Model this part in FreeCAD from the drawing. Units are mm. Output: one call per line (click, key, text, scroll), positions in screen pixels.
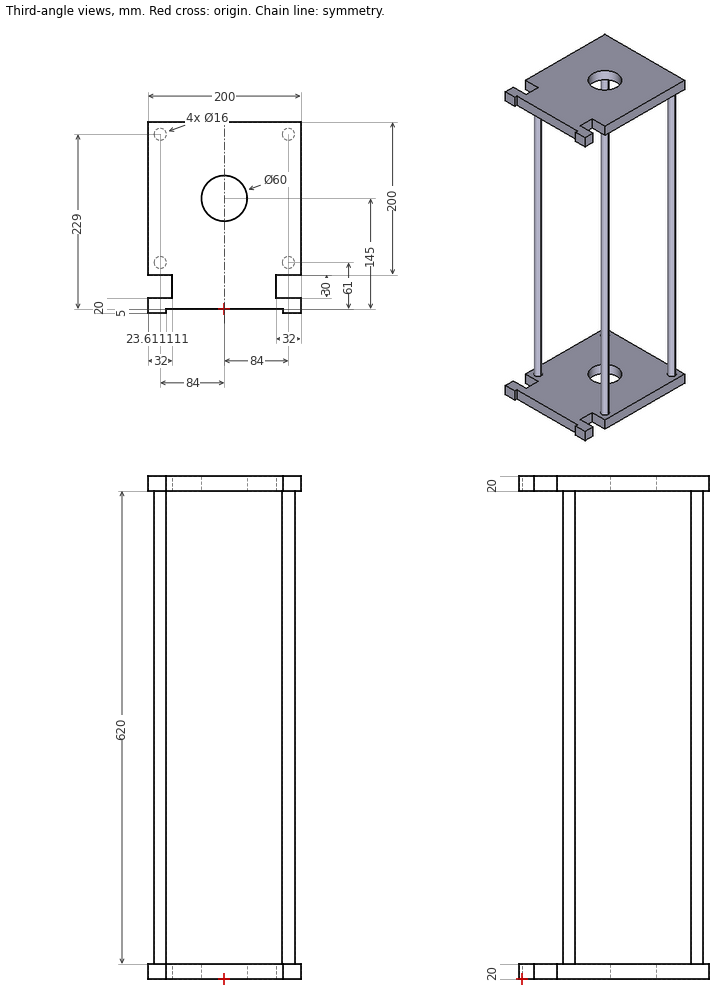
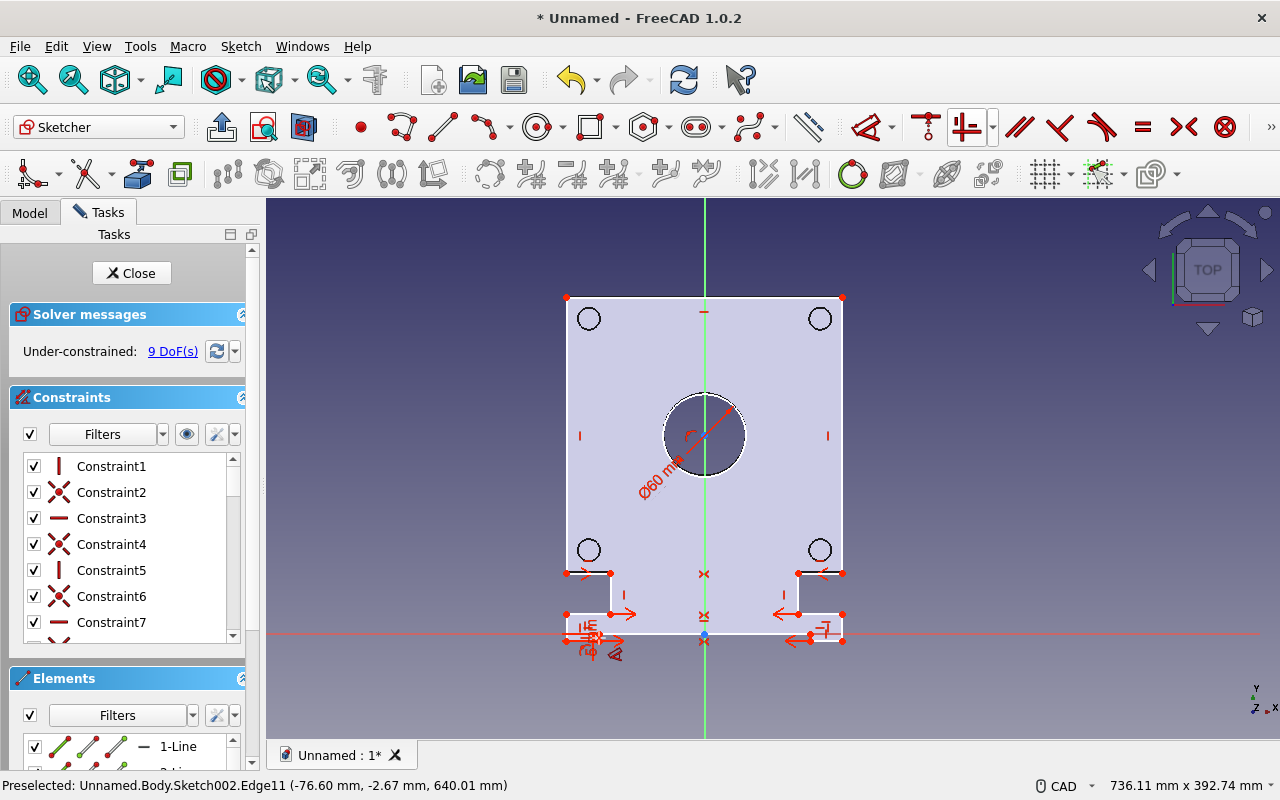
click(798, 602)
click(832, 594)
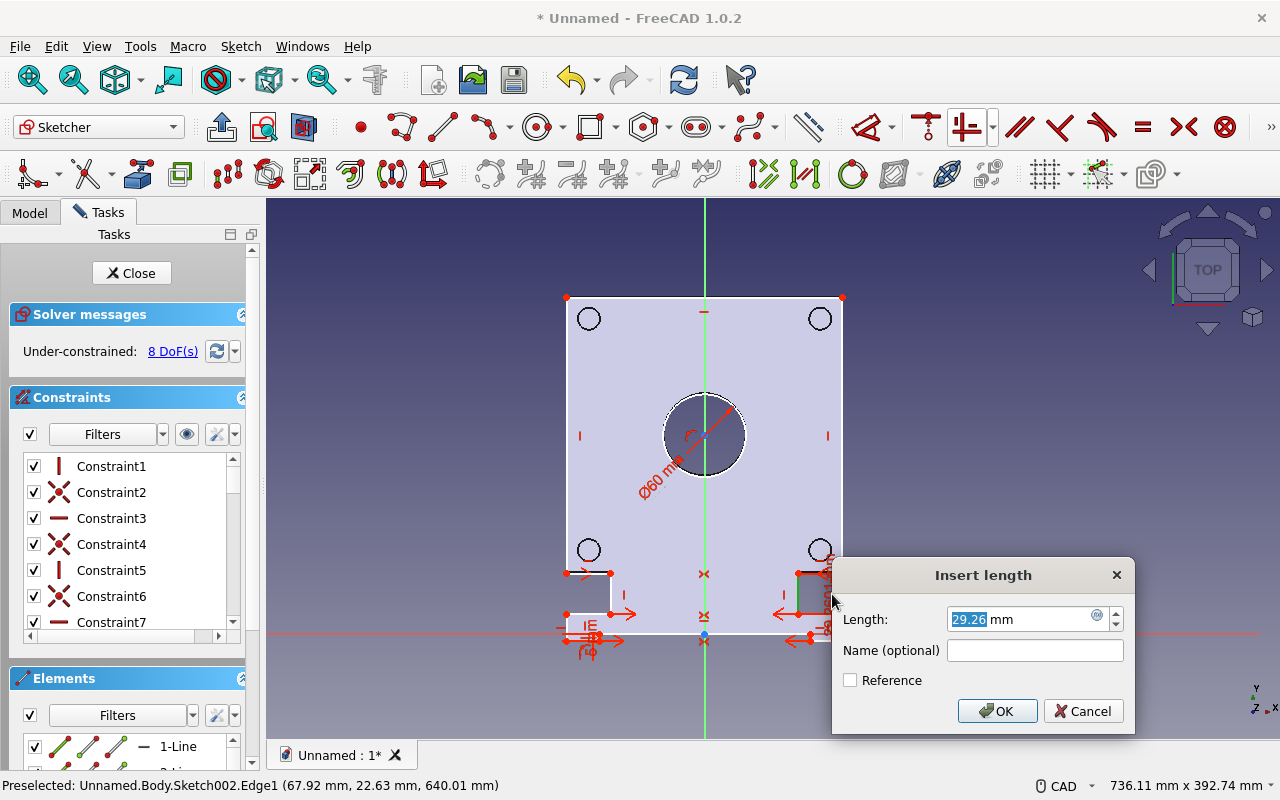
text(30)
key(Return)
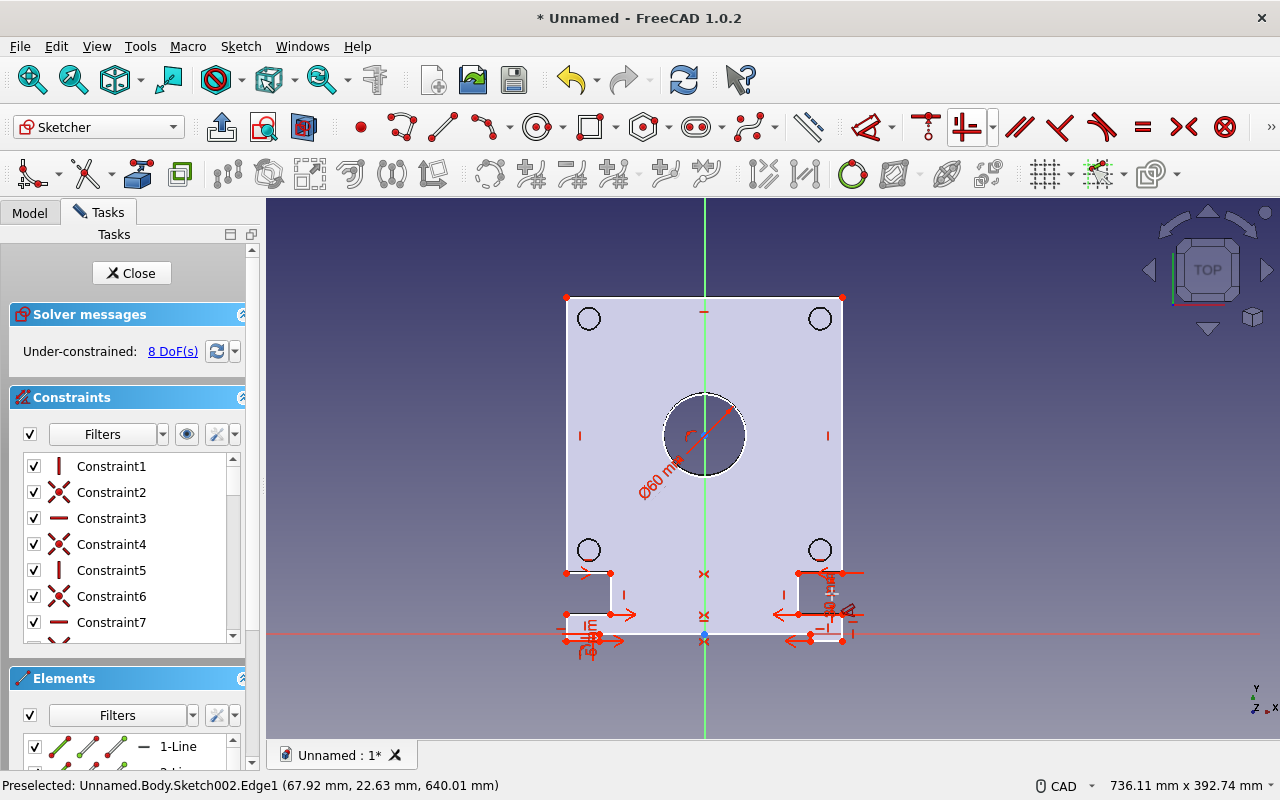
click(811, 573)
click(820, 539)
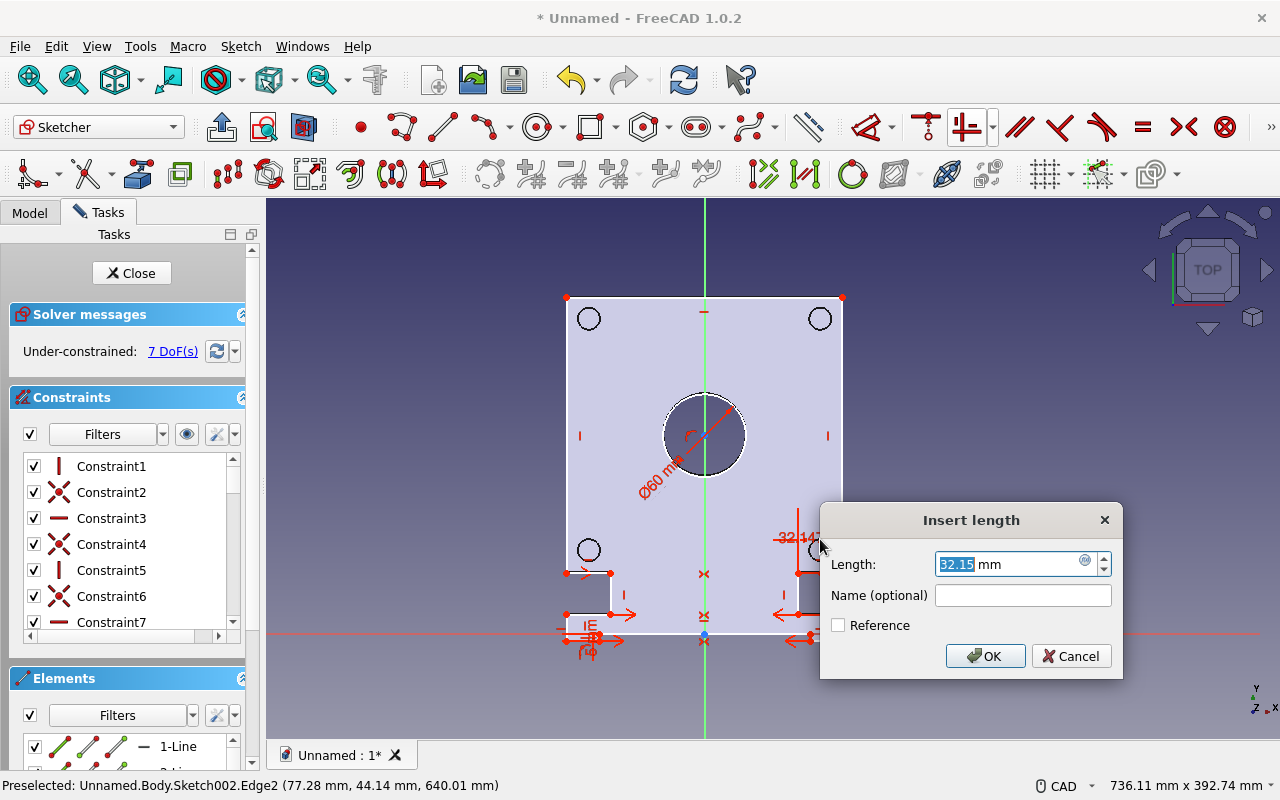
text(32)
key(Return)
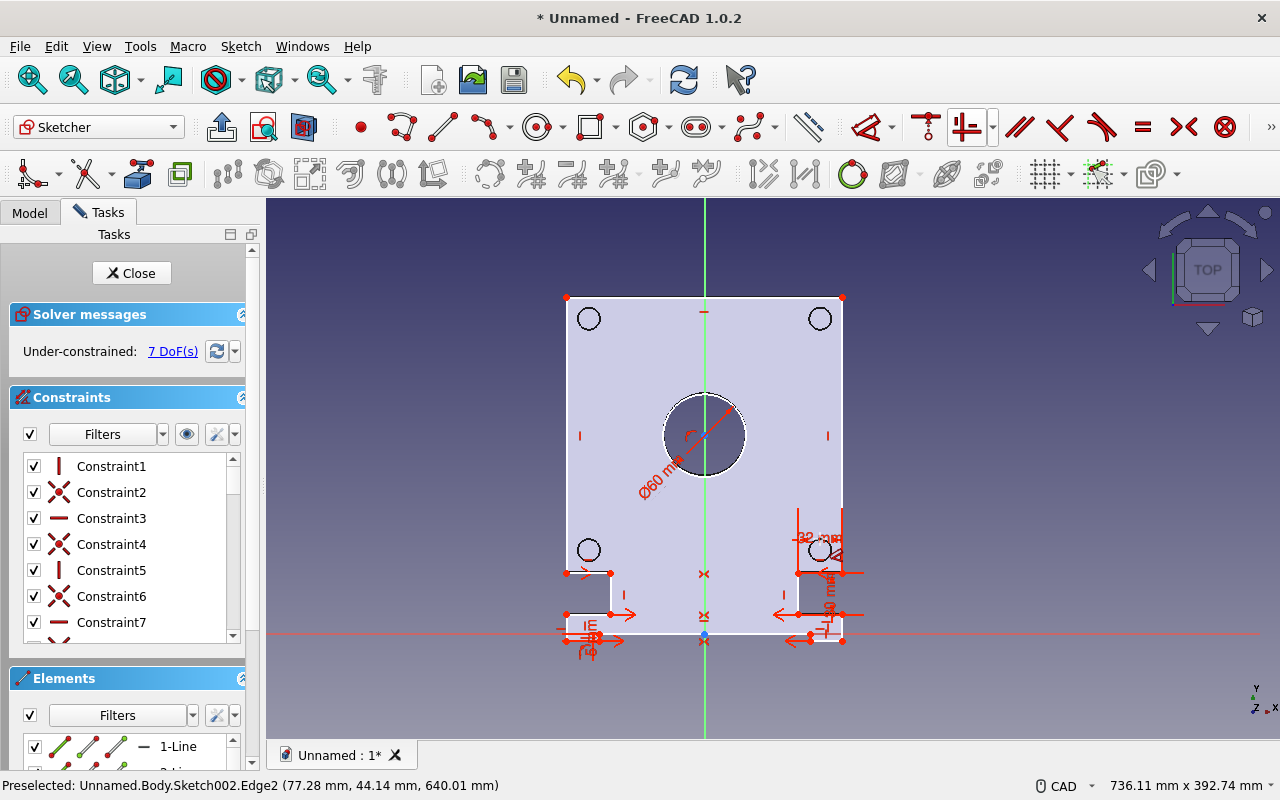
click(598, 615)
click(589, 673)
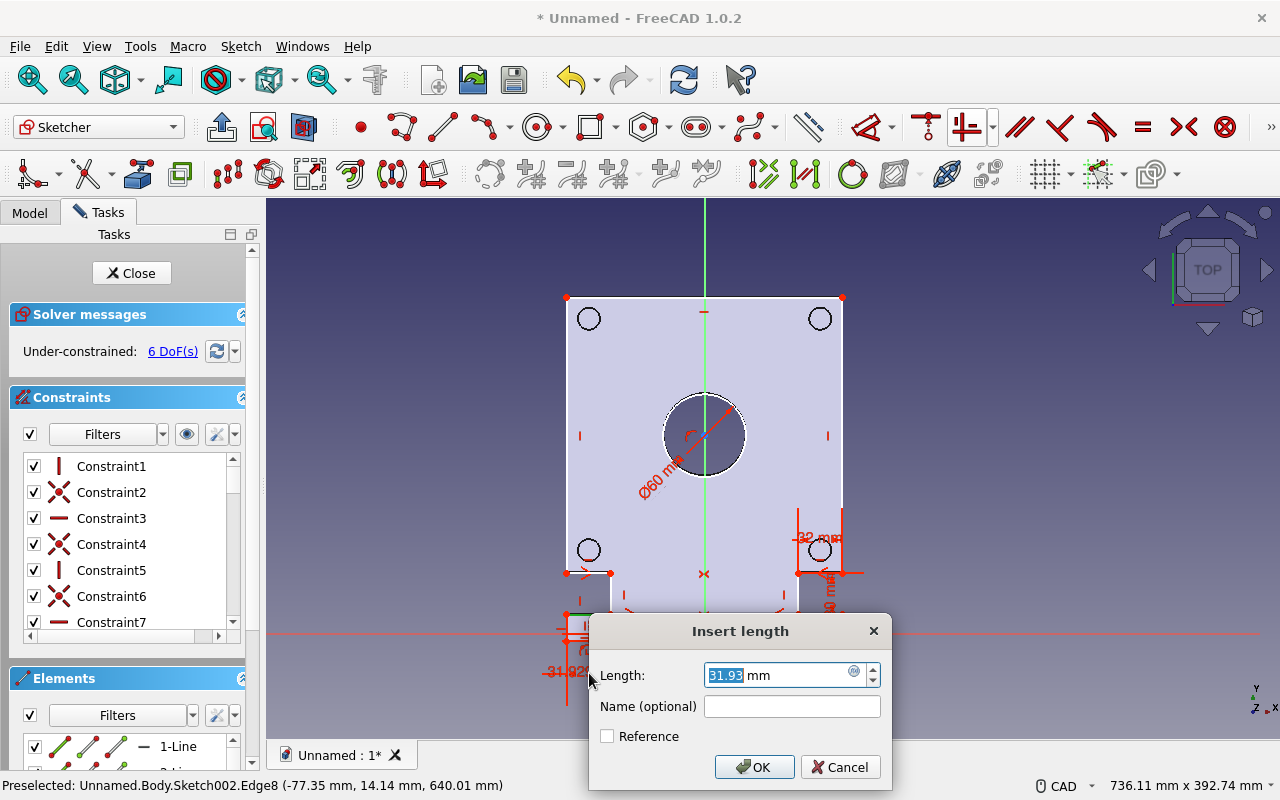
text(32)
key(Return)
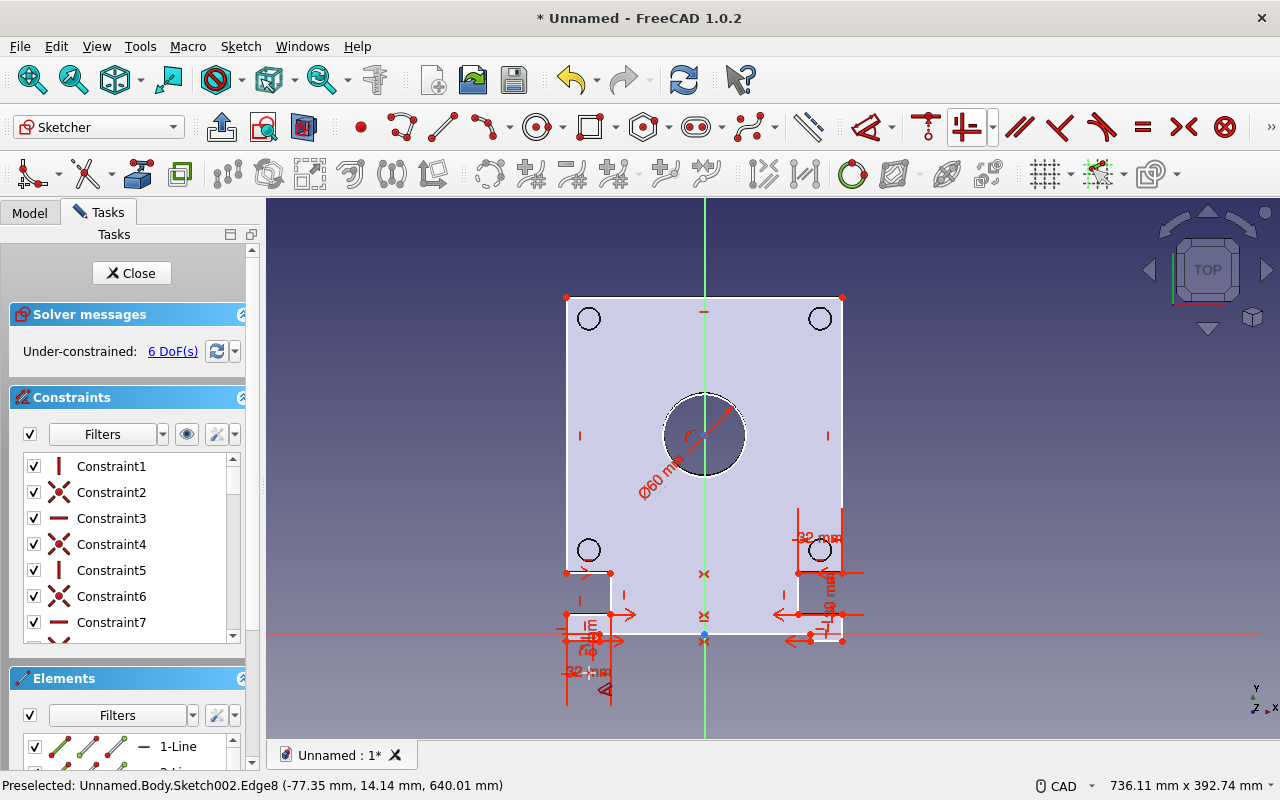
scroll(567, 631, up, 2)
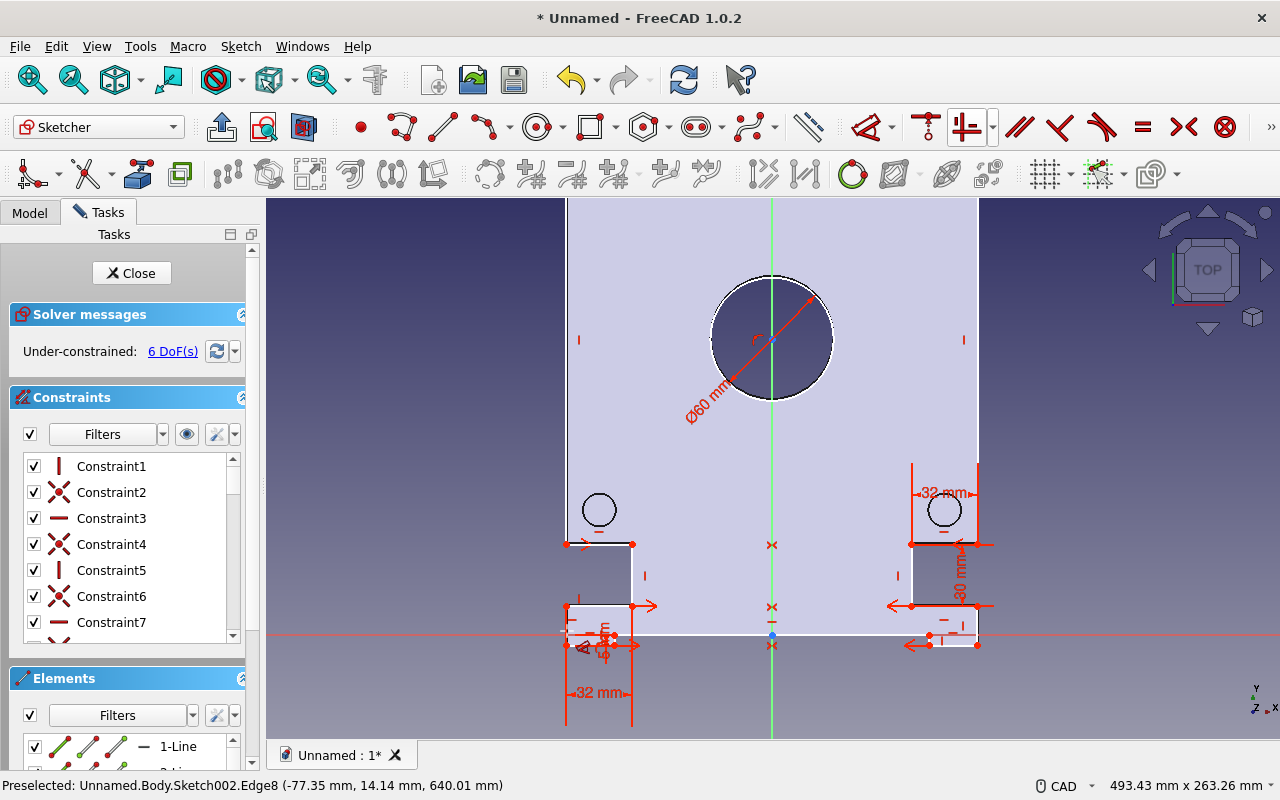
click(566, 630)
click(532, 617)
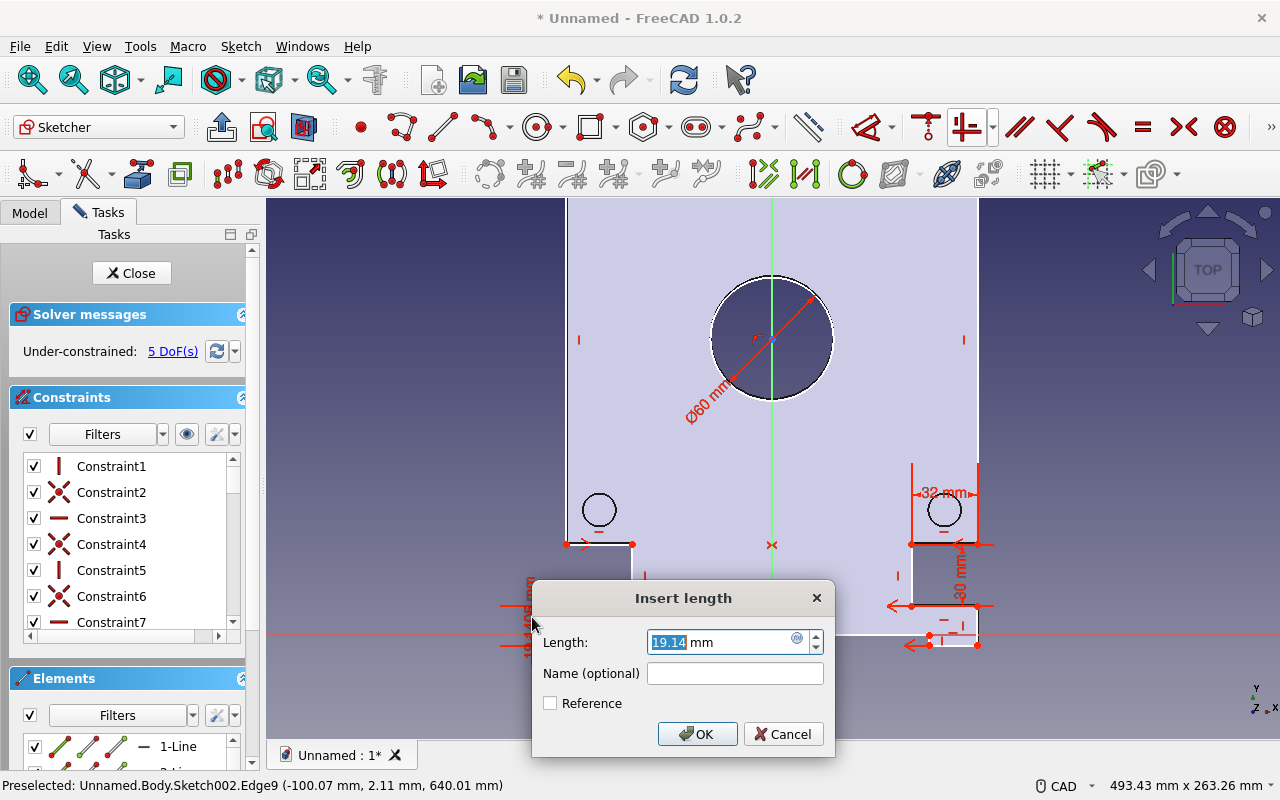
text(20)
key(Return)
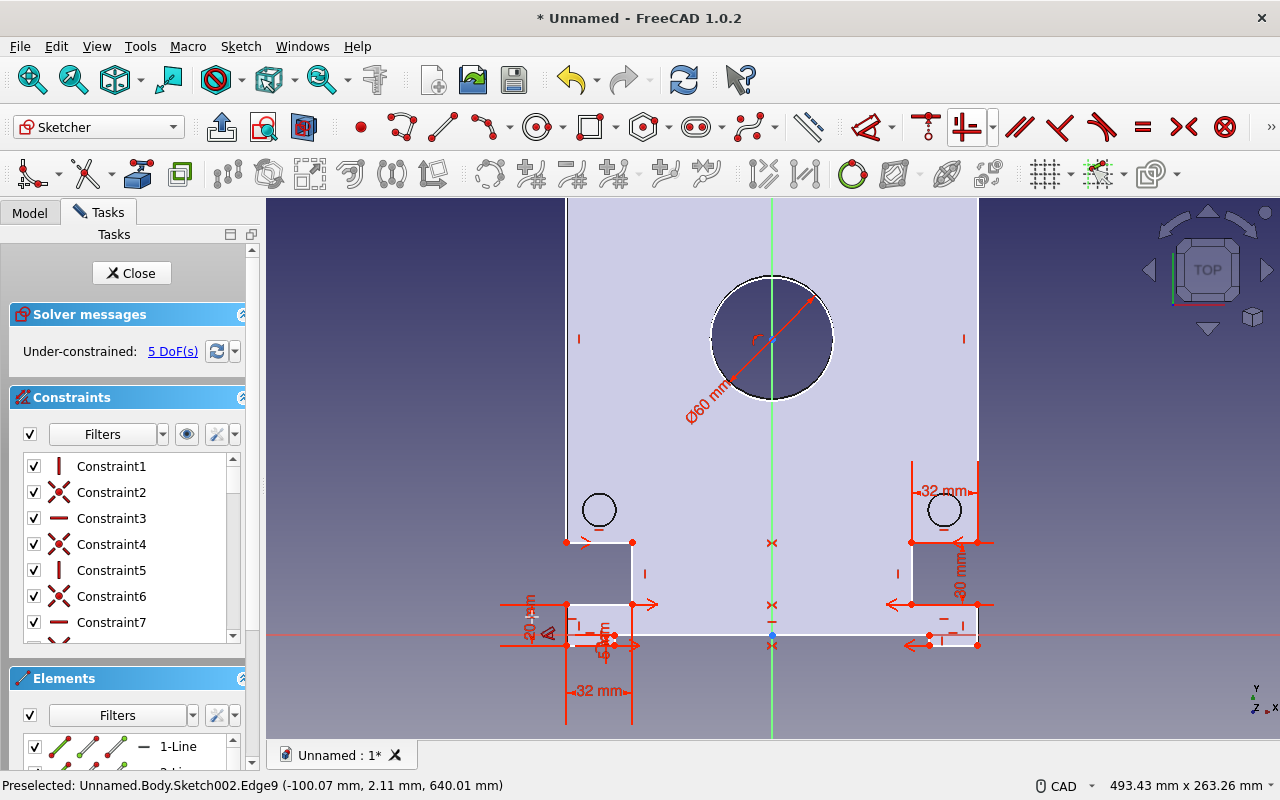
click(958, 605)
click(945, 663)